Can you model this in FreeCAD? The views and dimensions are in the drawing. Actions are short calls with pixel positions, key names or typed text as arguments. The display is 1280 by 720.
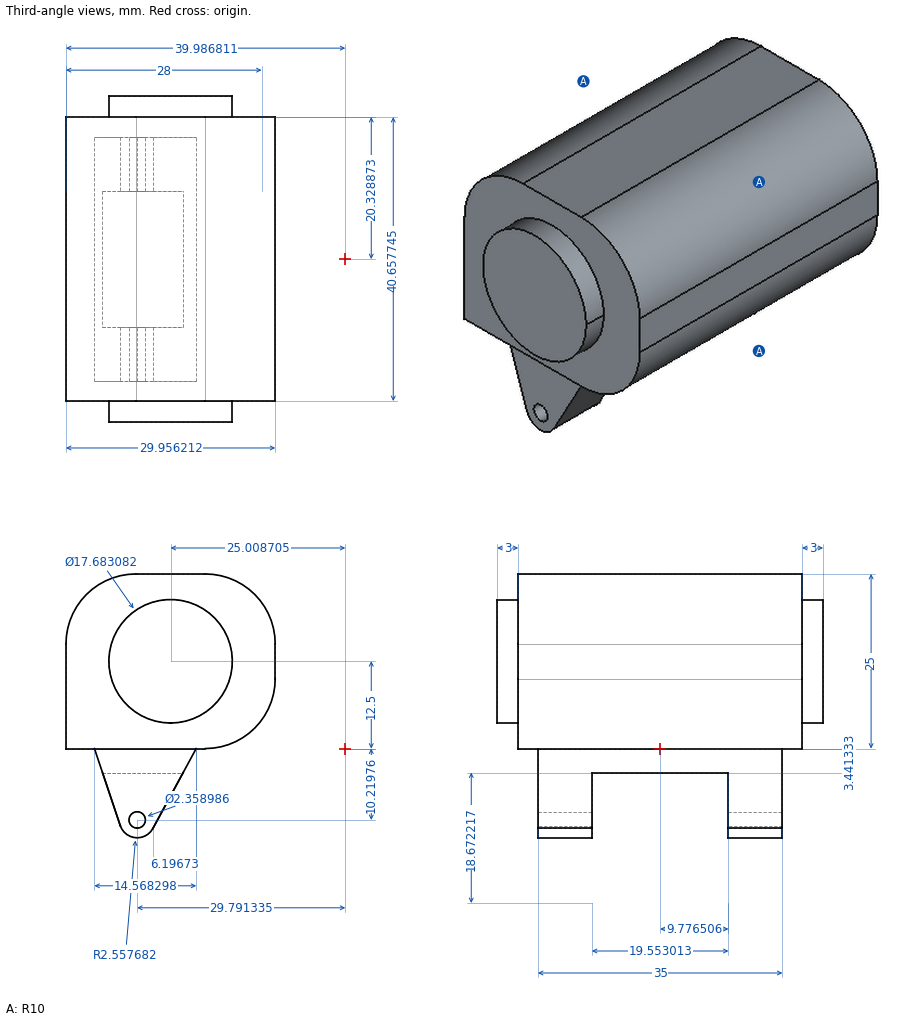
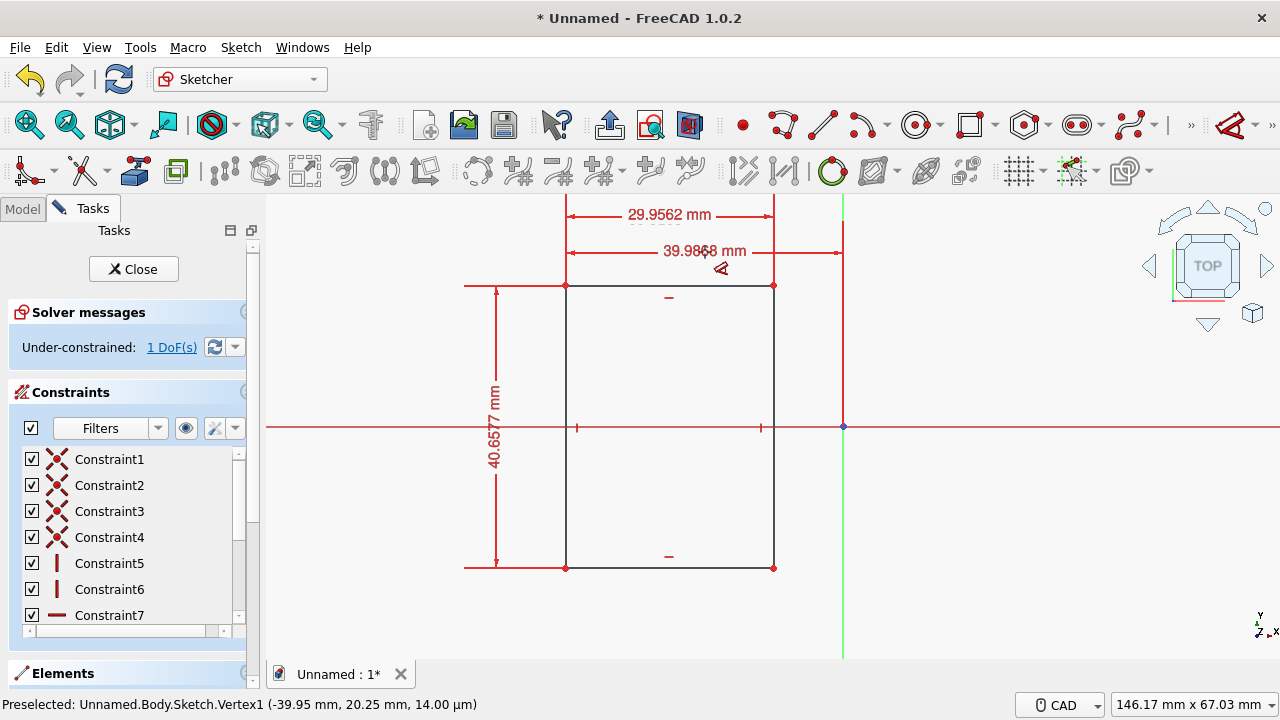
click(566, 286)
click(532, 356)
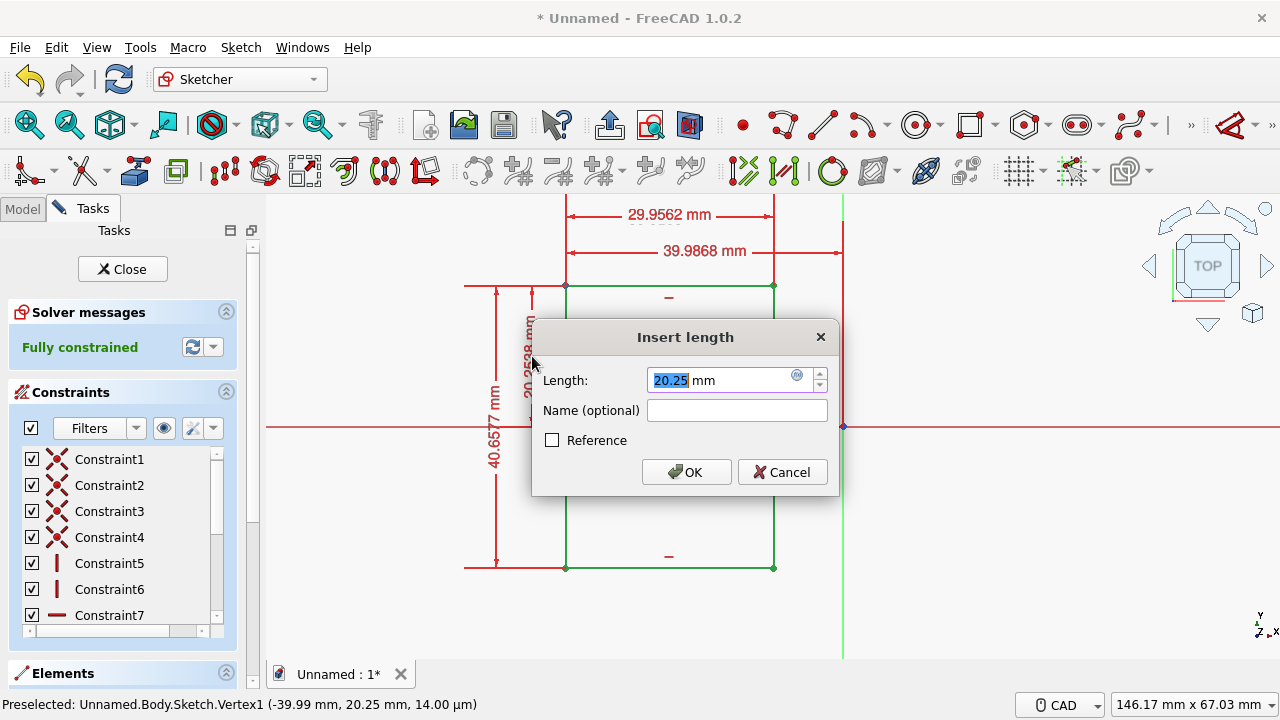
text(20.328873)
key(Return)
key(Escape)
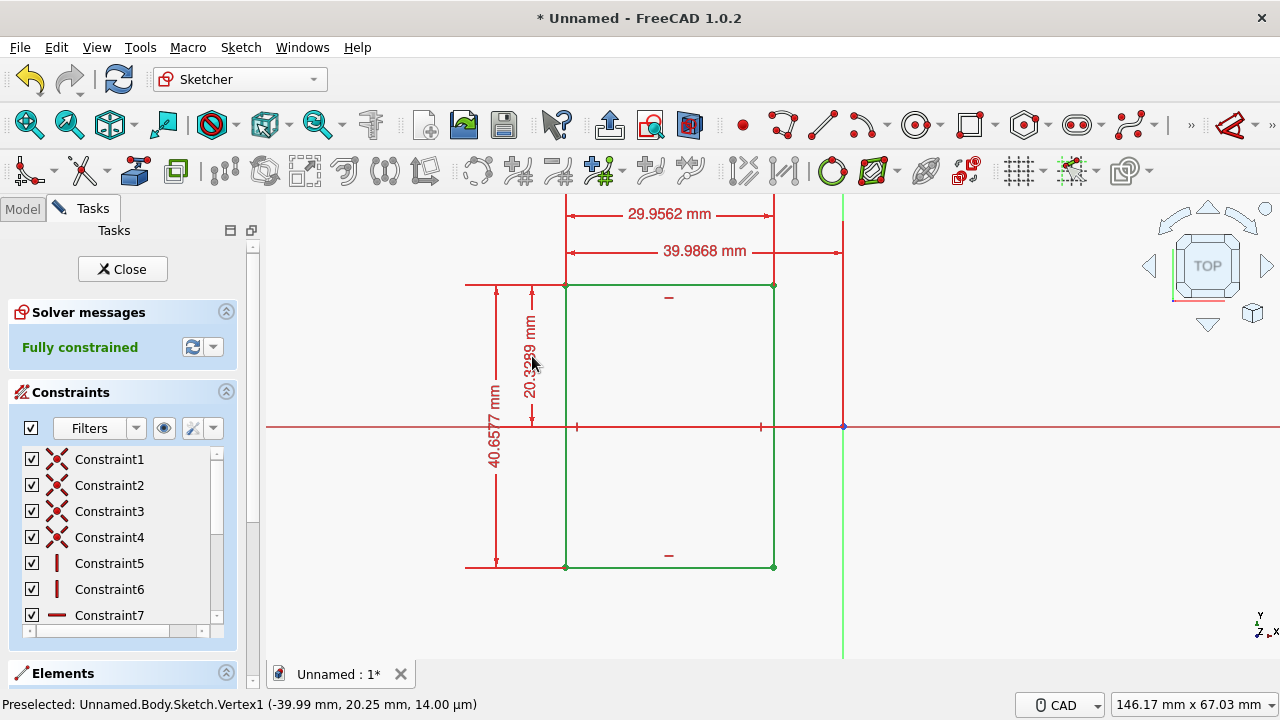
click(123, 269)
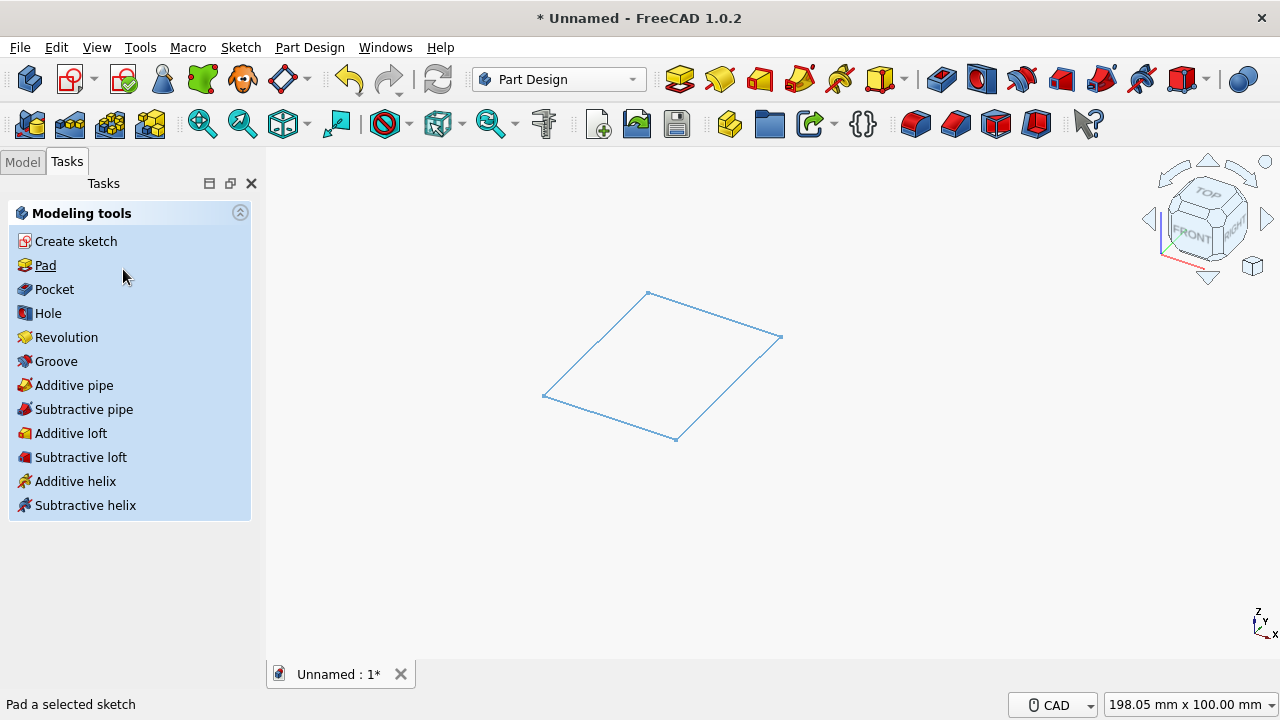
click(680, 80)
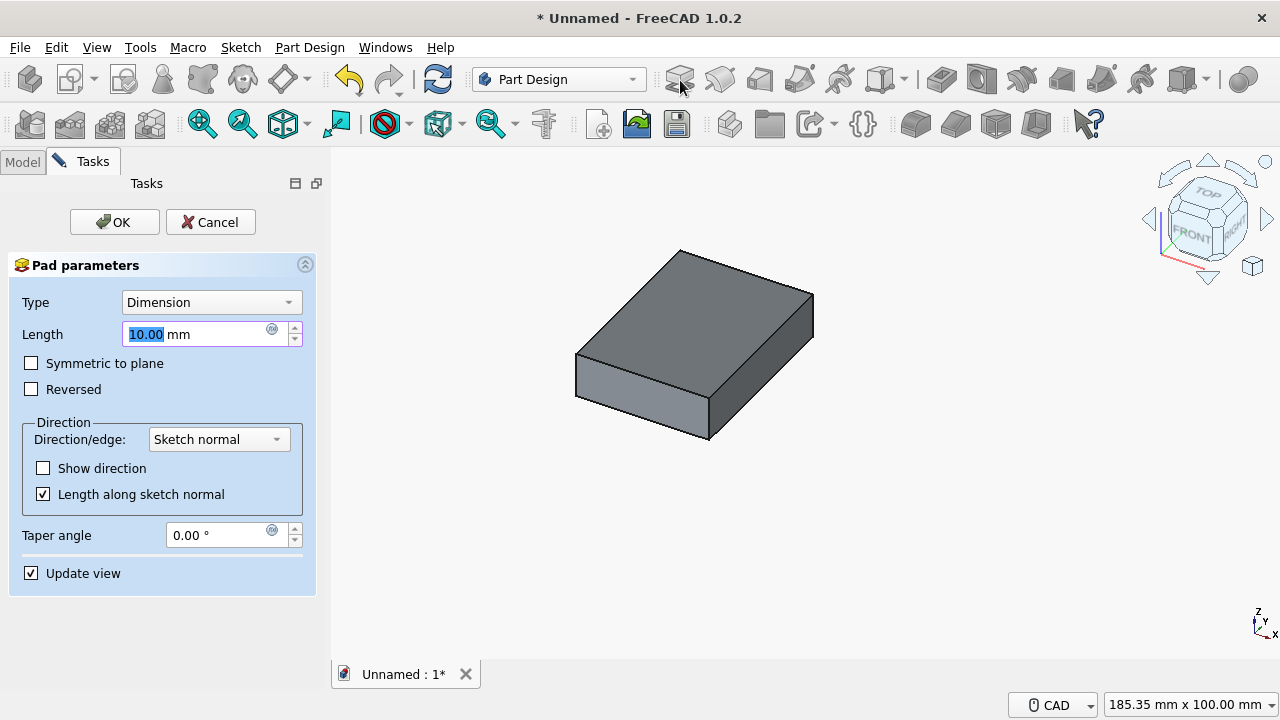
text(25)
key(Tab)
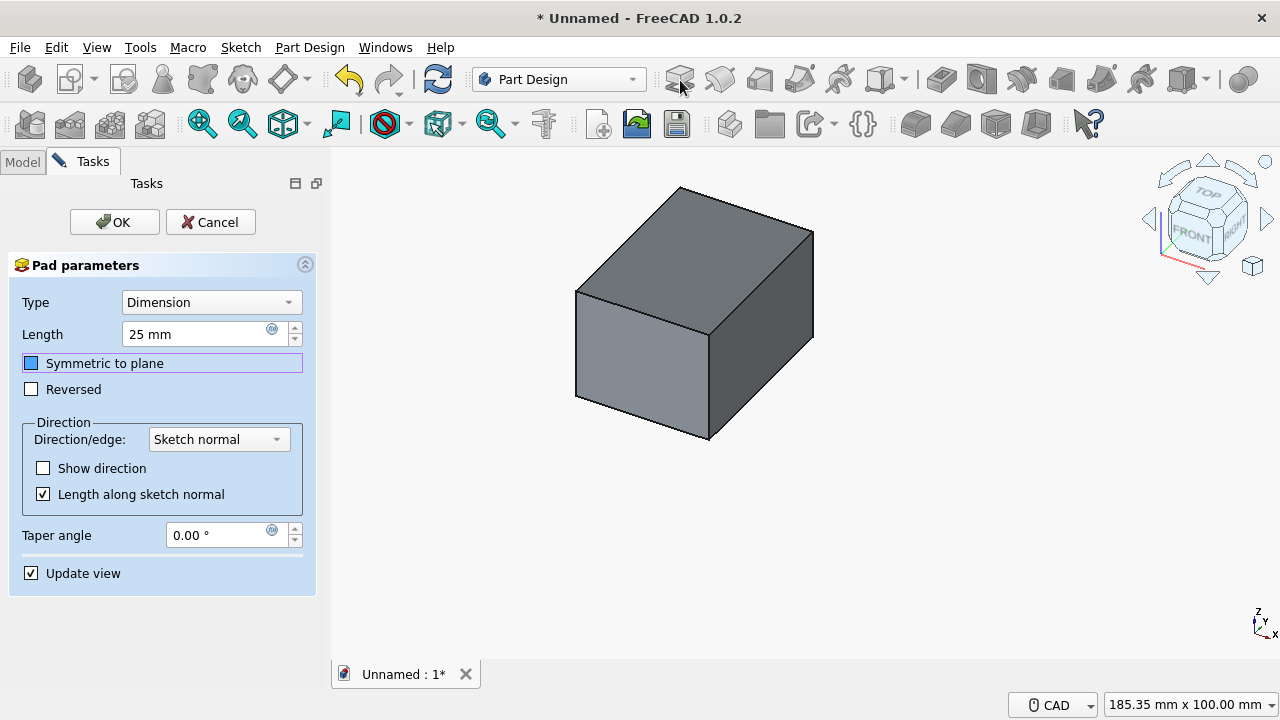
click(115, 222)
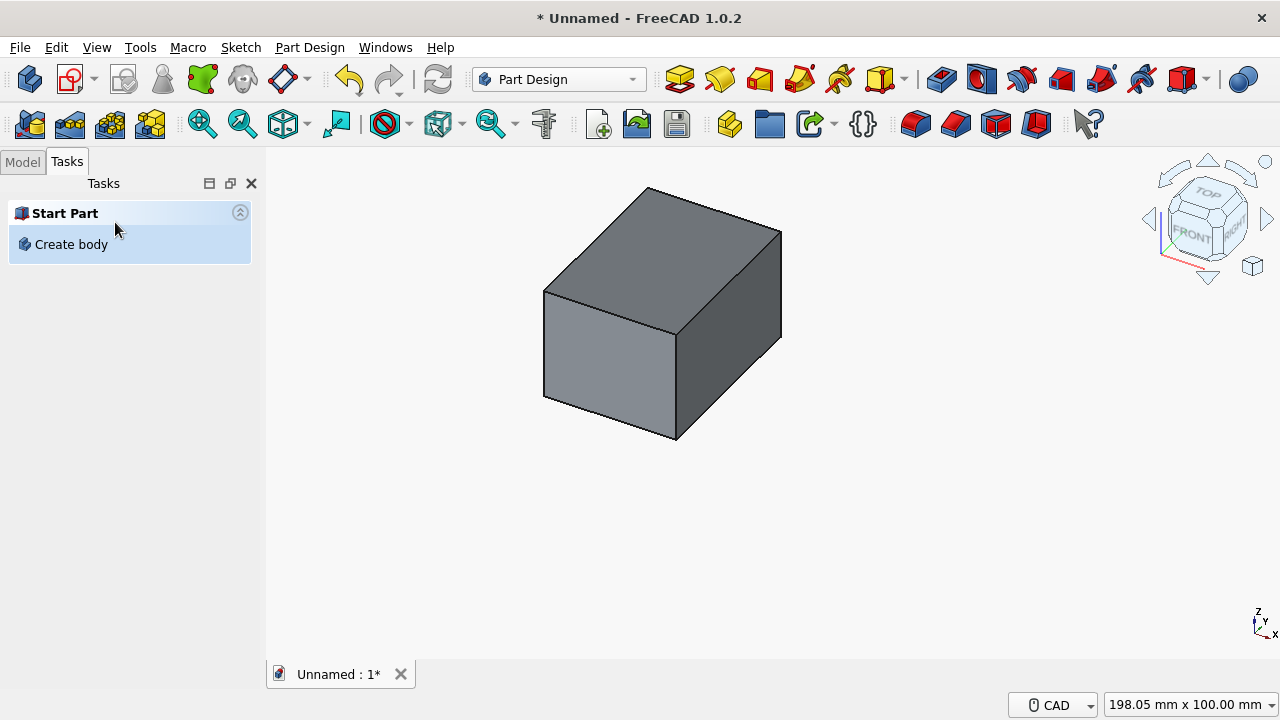
click(70, 80)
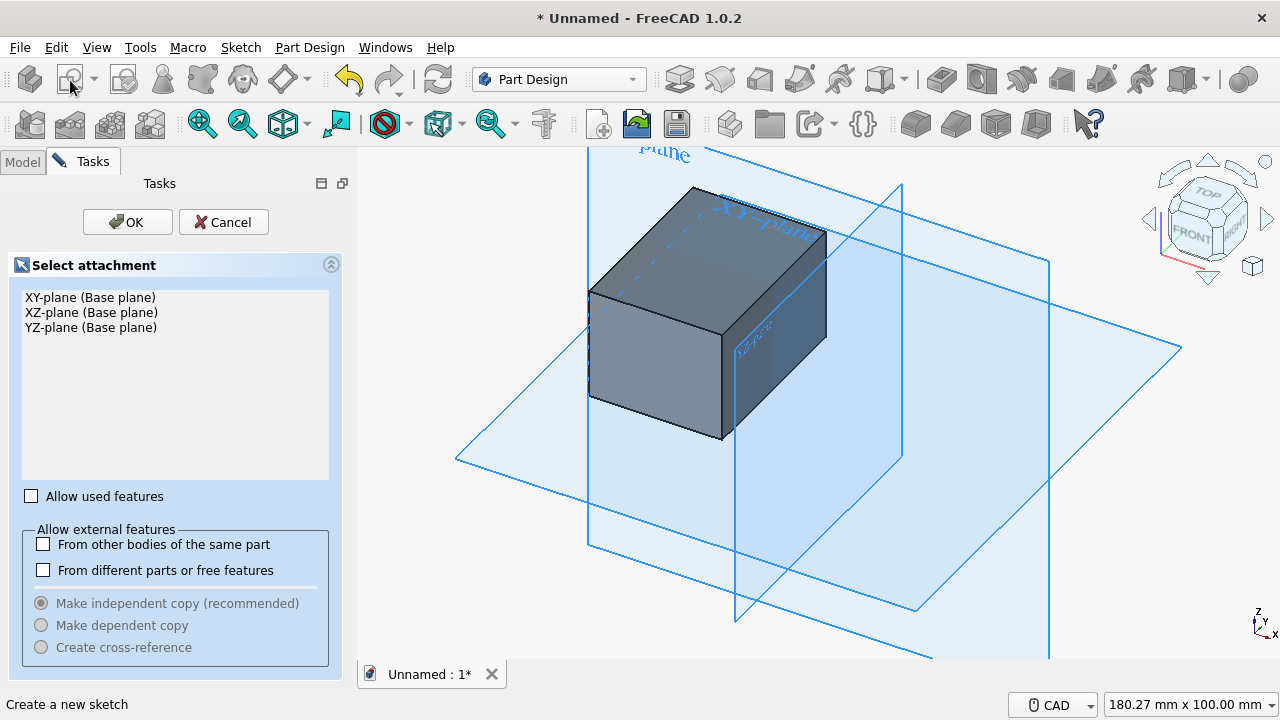
click(82, 312)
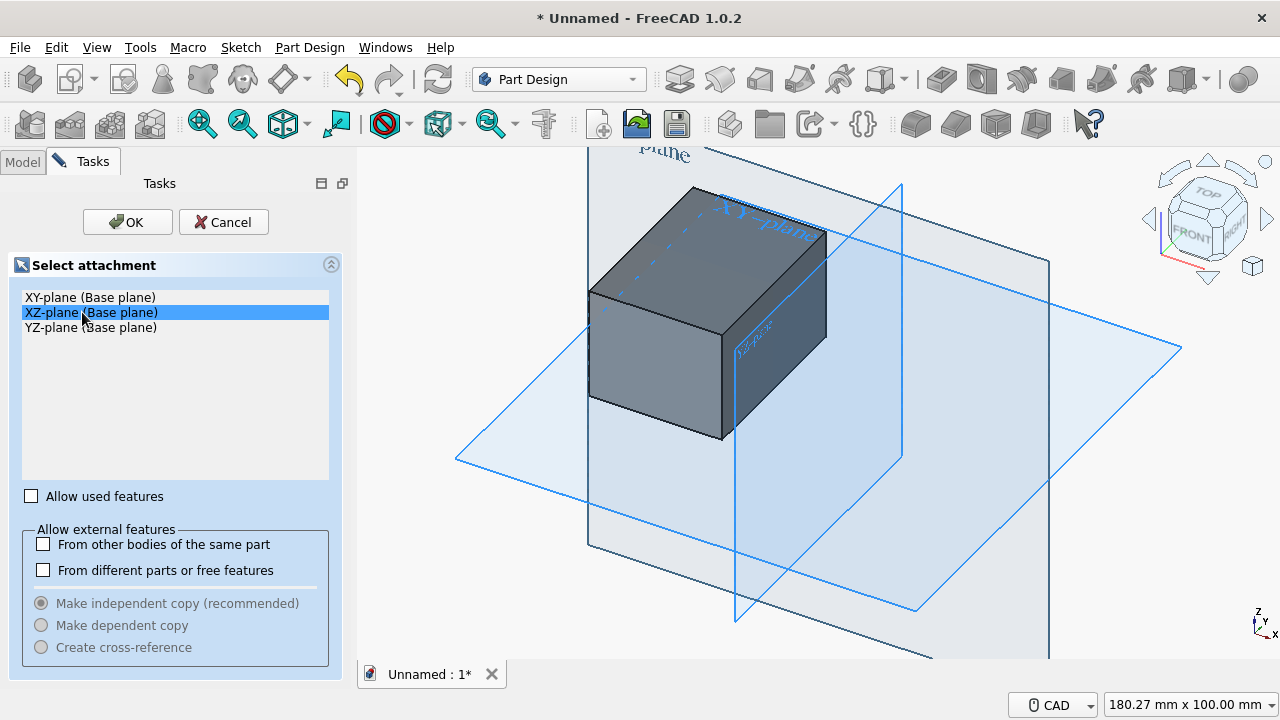
click(128, 222)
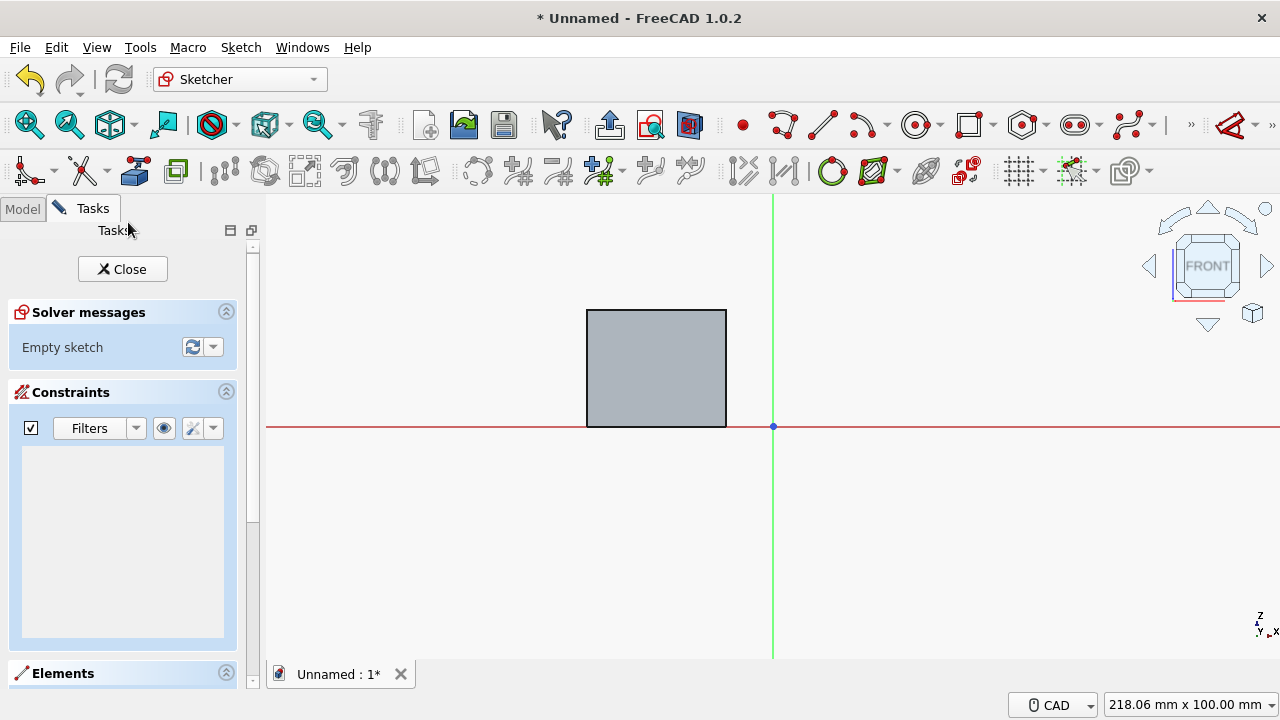
click(690, 126)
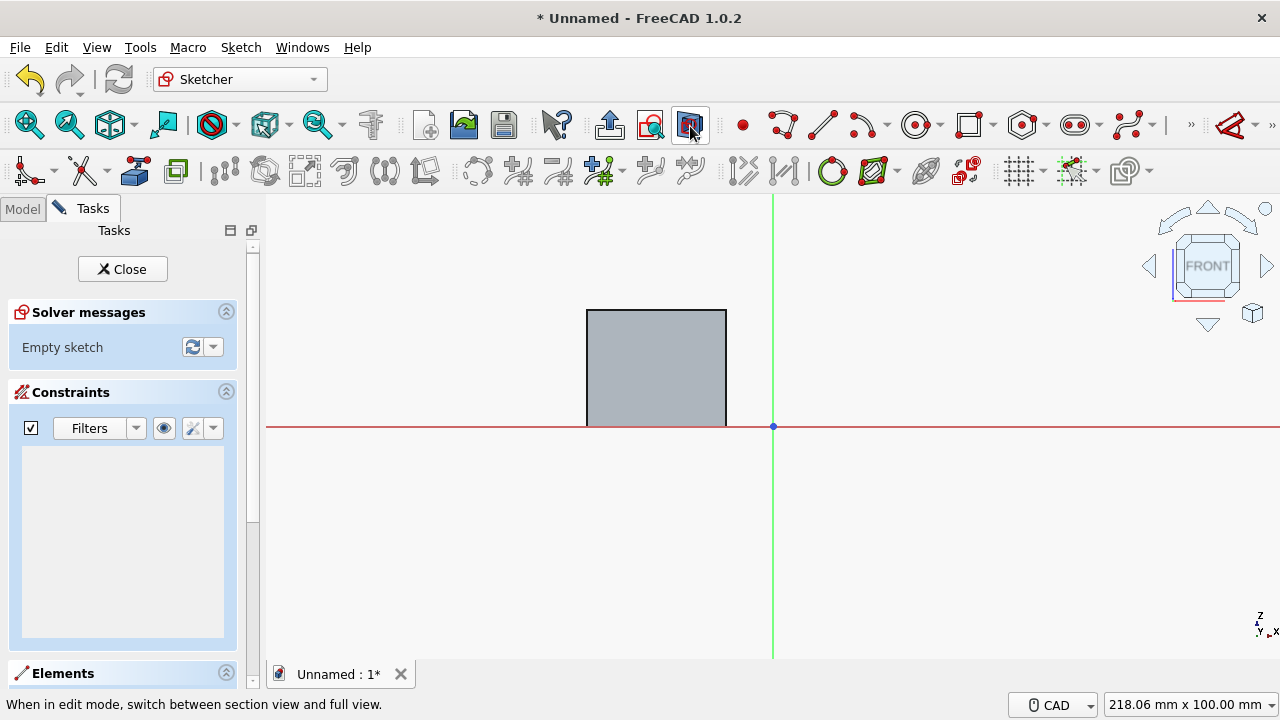
scroll(683, 469, up, 6)